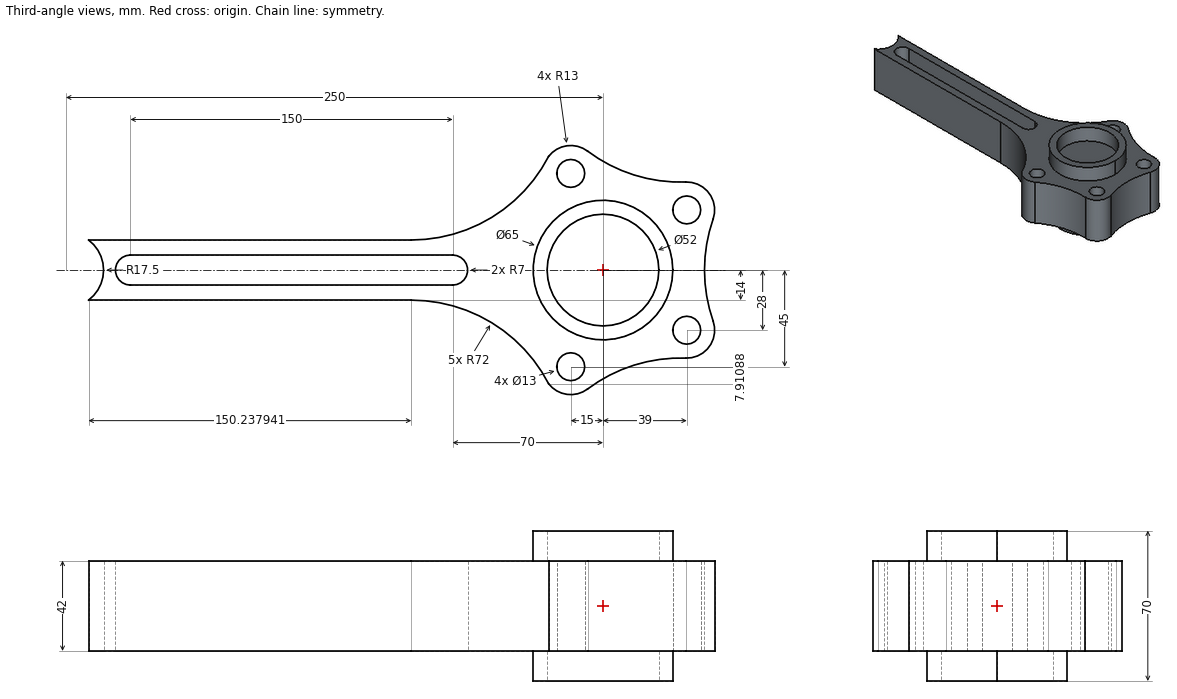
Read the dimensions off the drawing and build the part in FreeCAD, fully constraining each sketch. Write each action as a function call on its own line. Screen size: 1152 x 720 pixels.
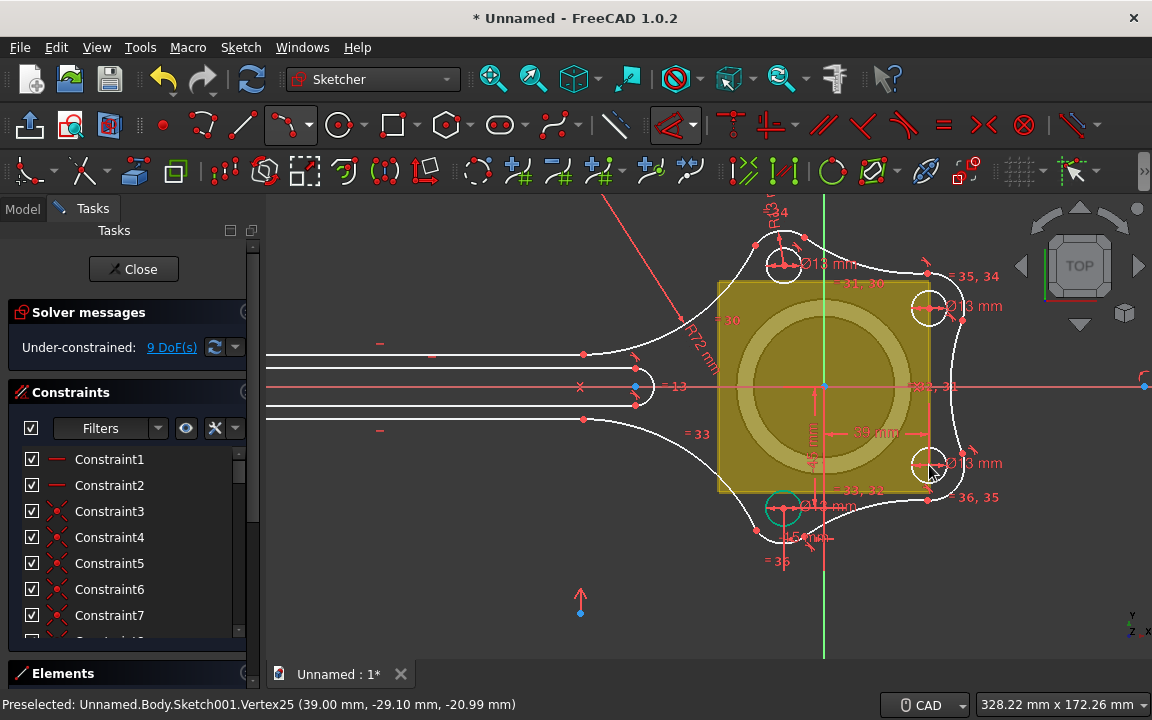
click(696, 126)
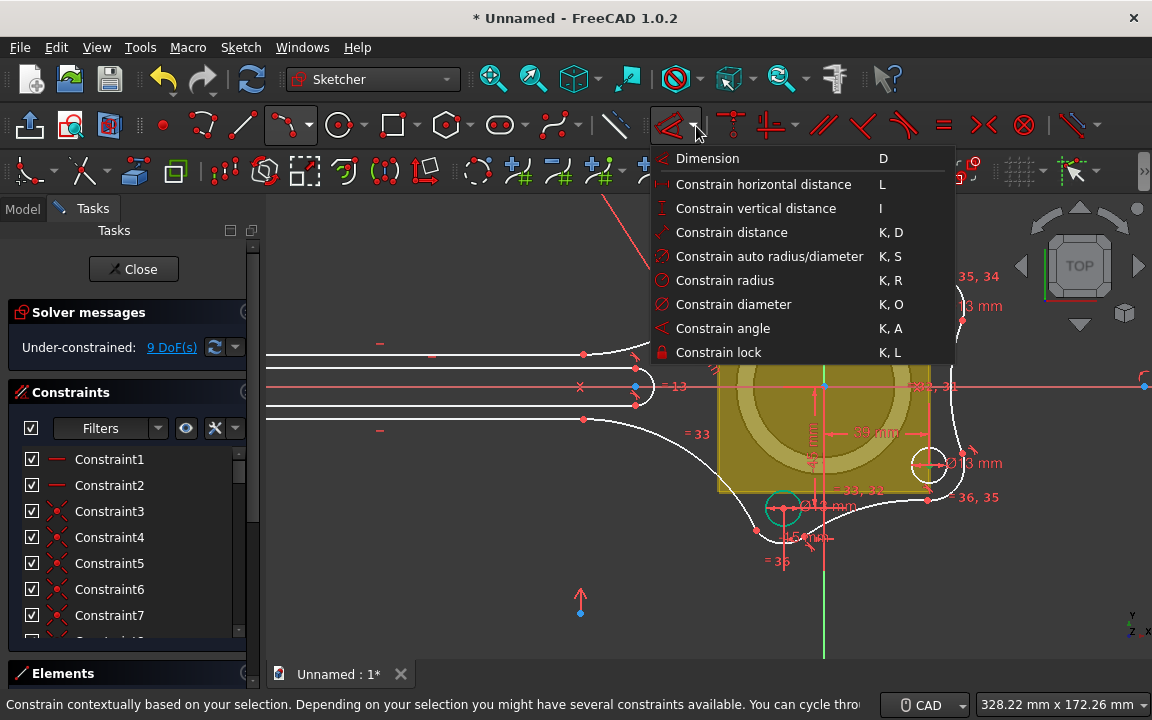
click(803, 208)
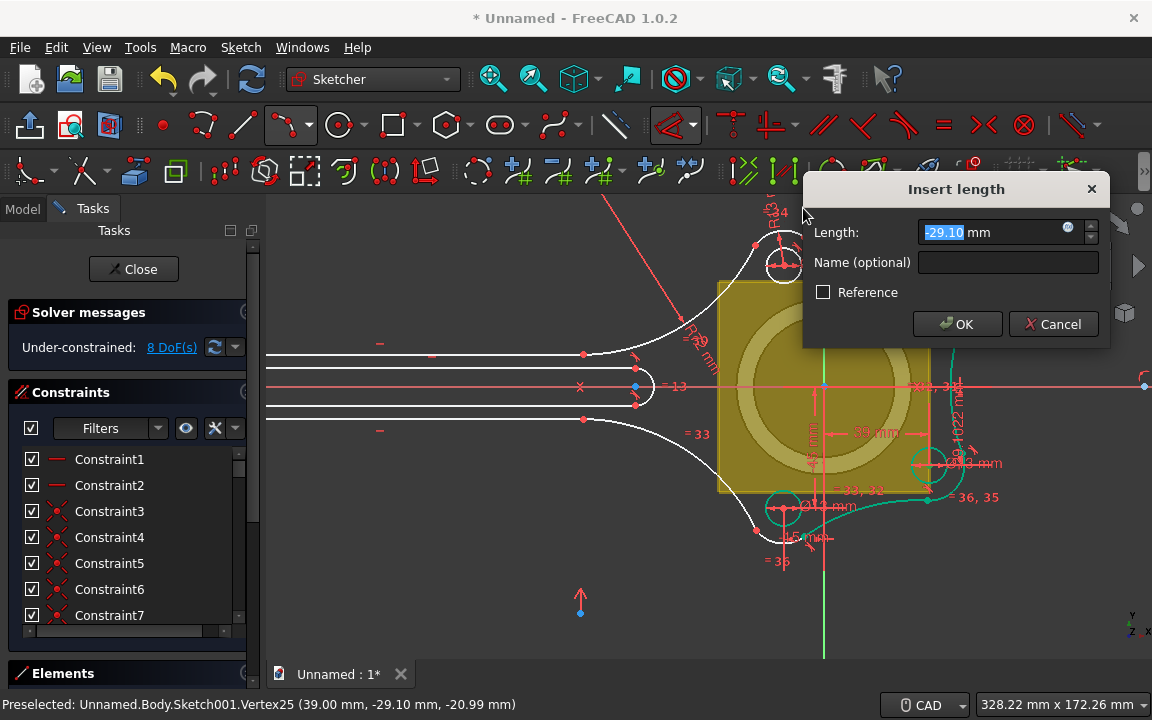
text(-28)
key(Return)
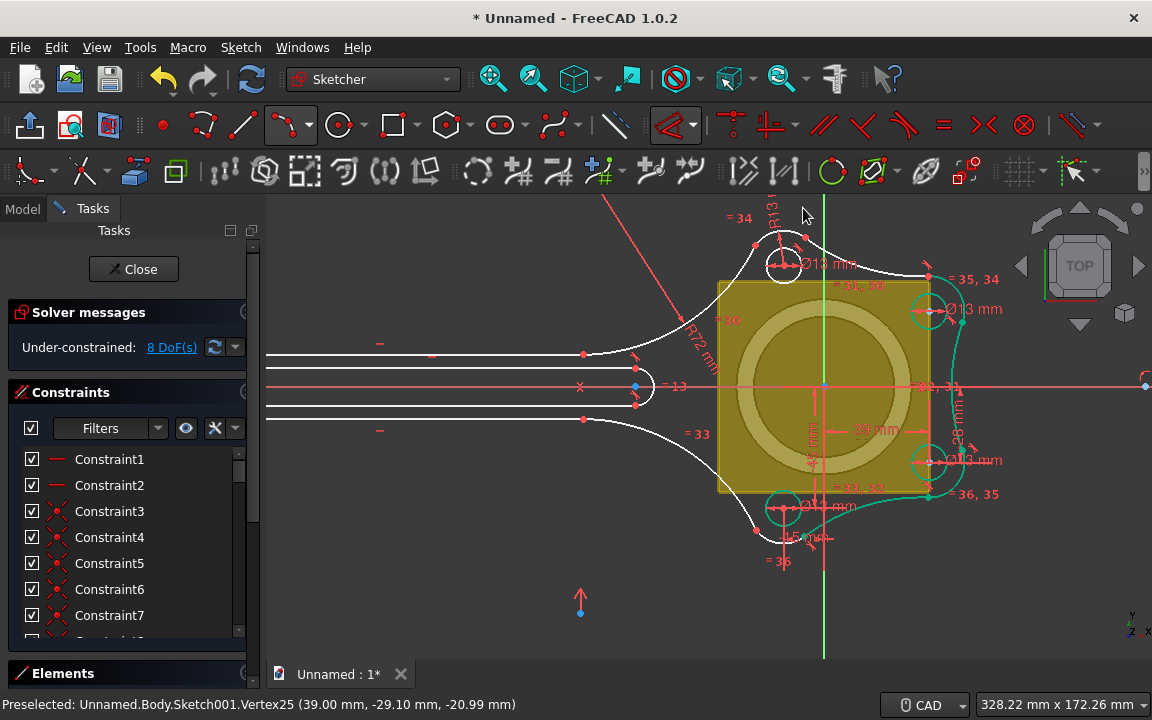
click(784, 266)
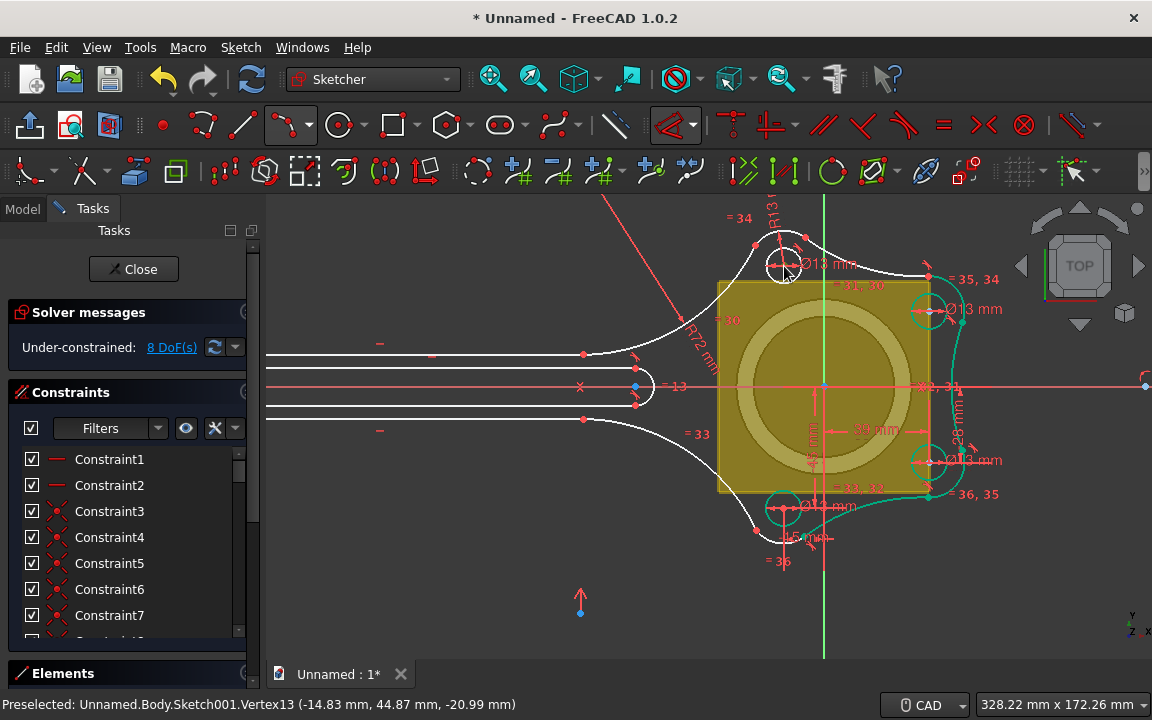
key(l)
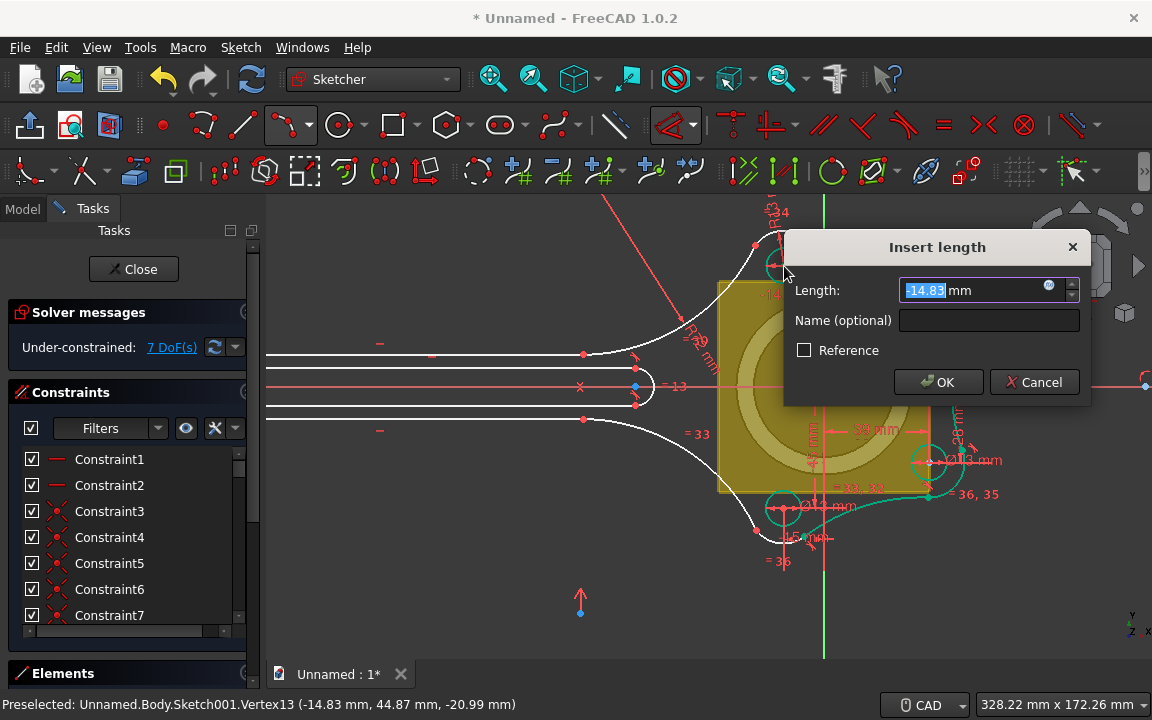
text(-15)
key(Return)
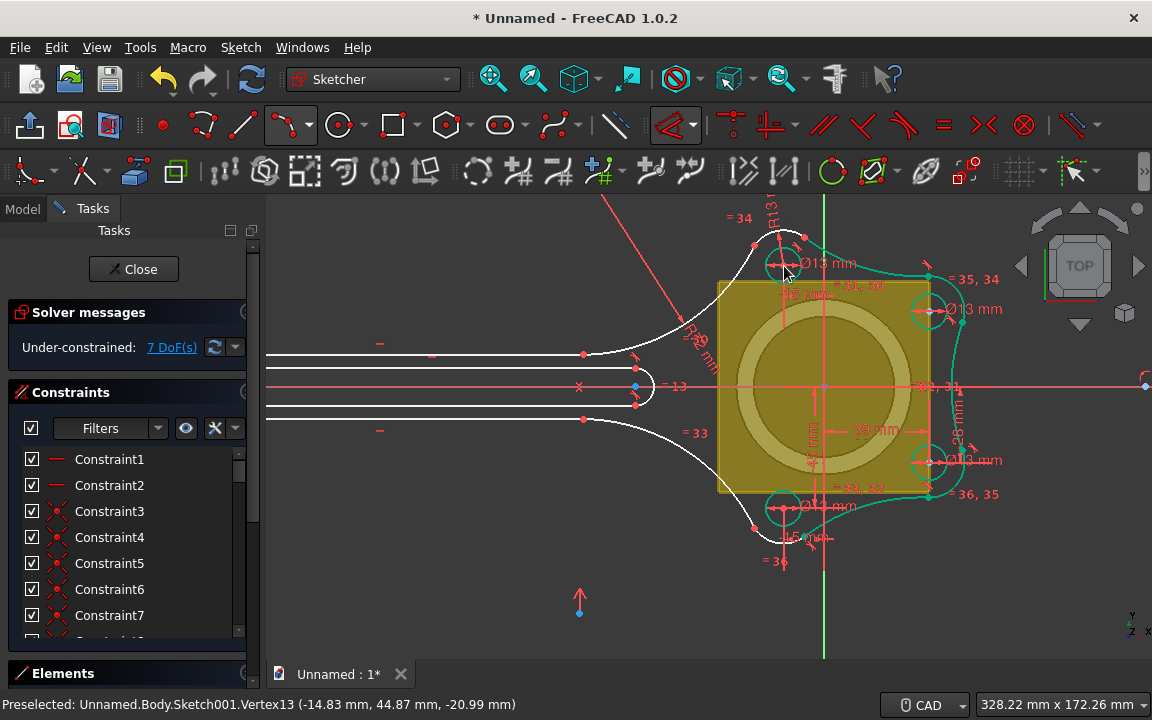
click(352, 368)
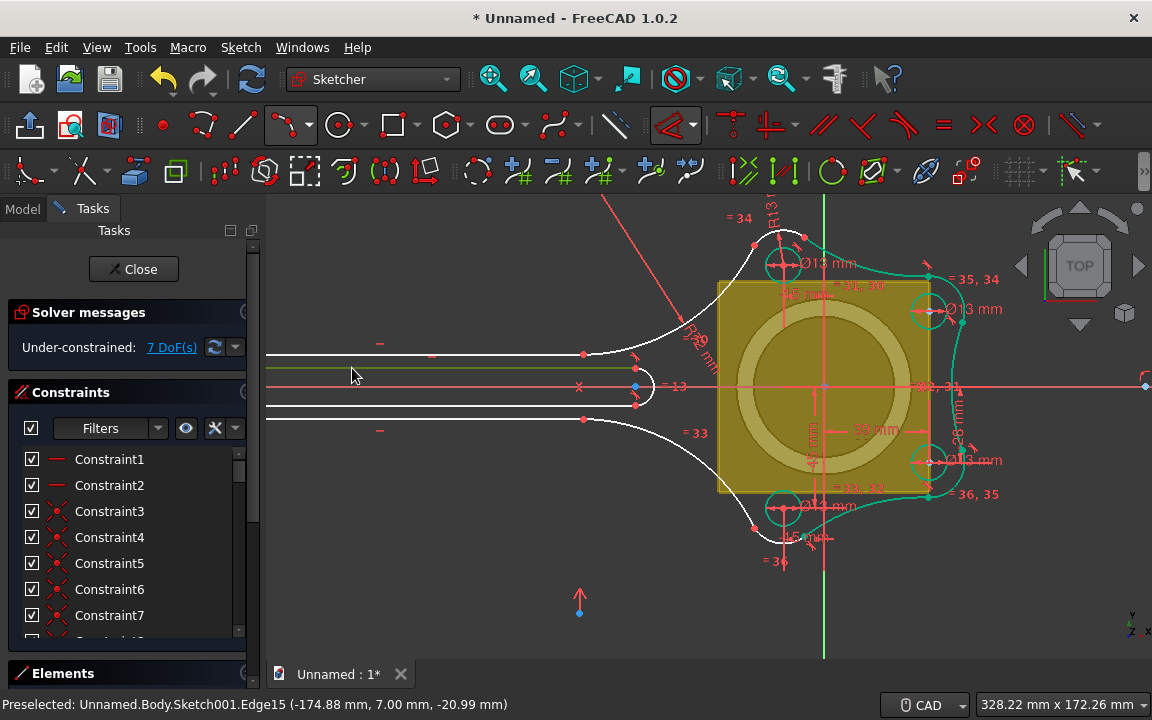
key(l)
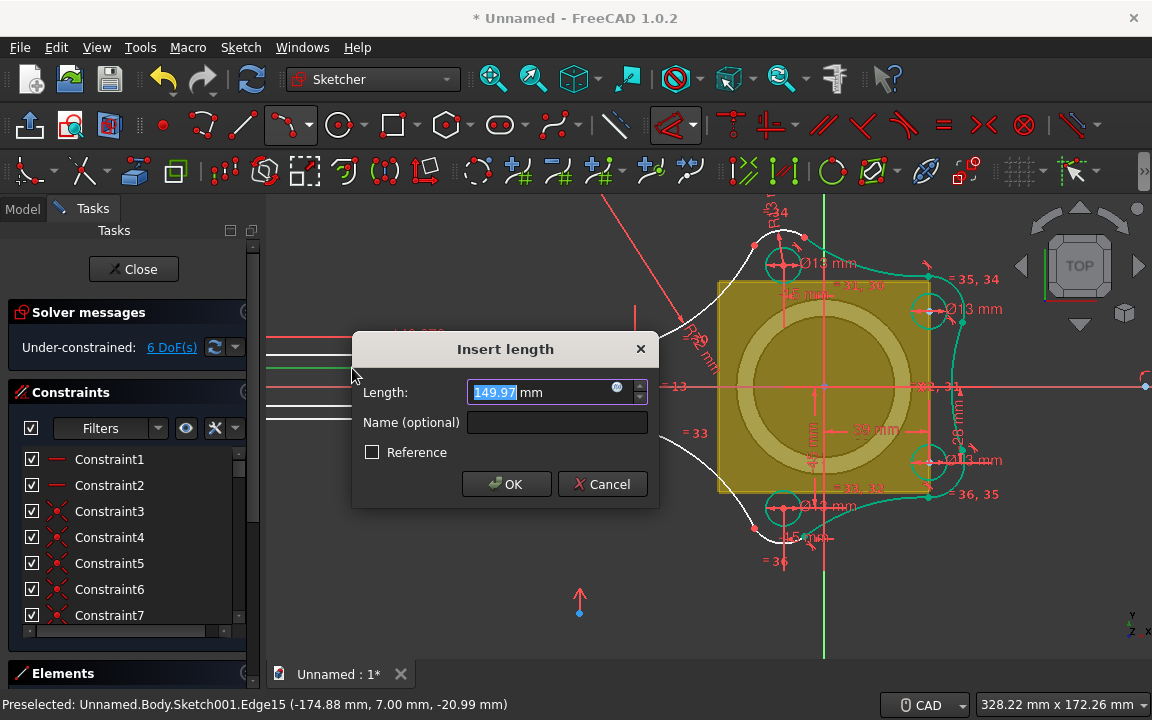
text(150)
key(Return)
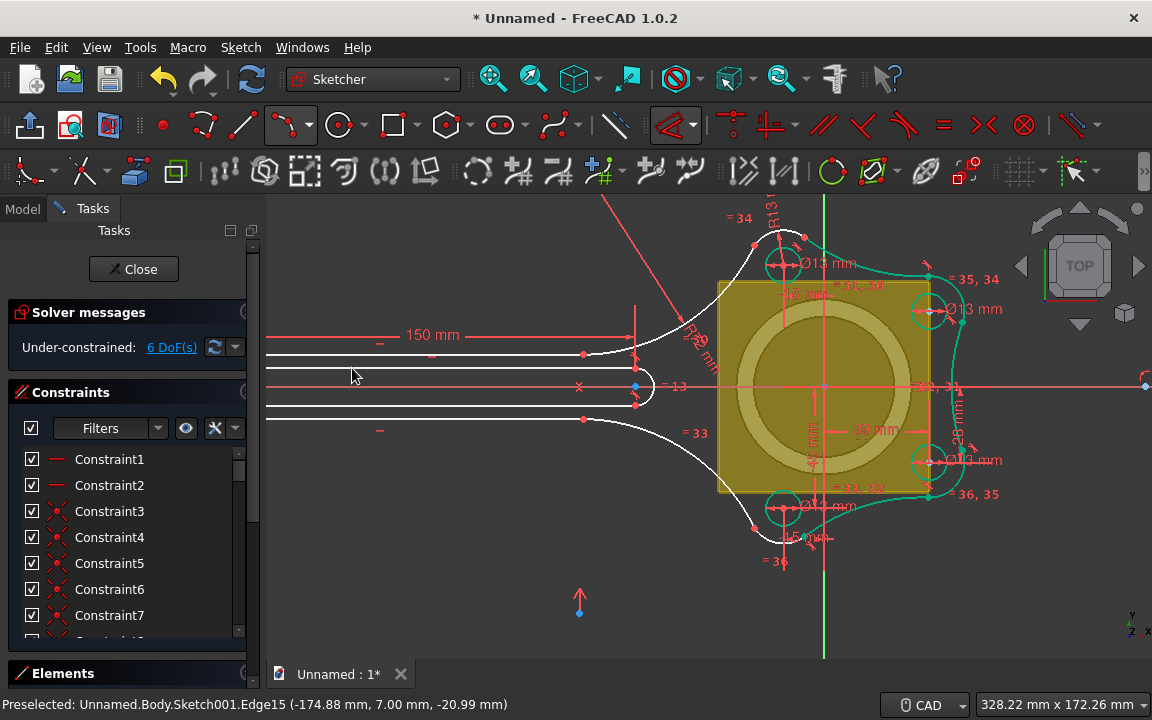
click(584, 419)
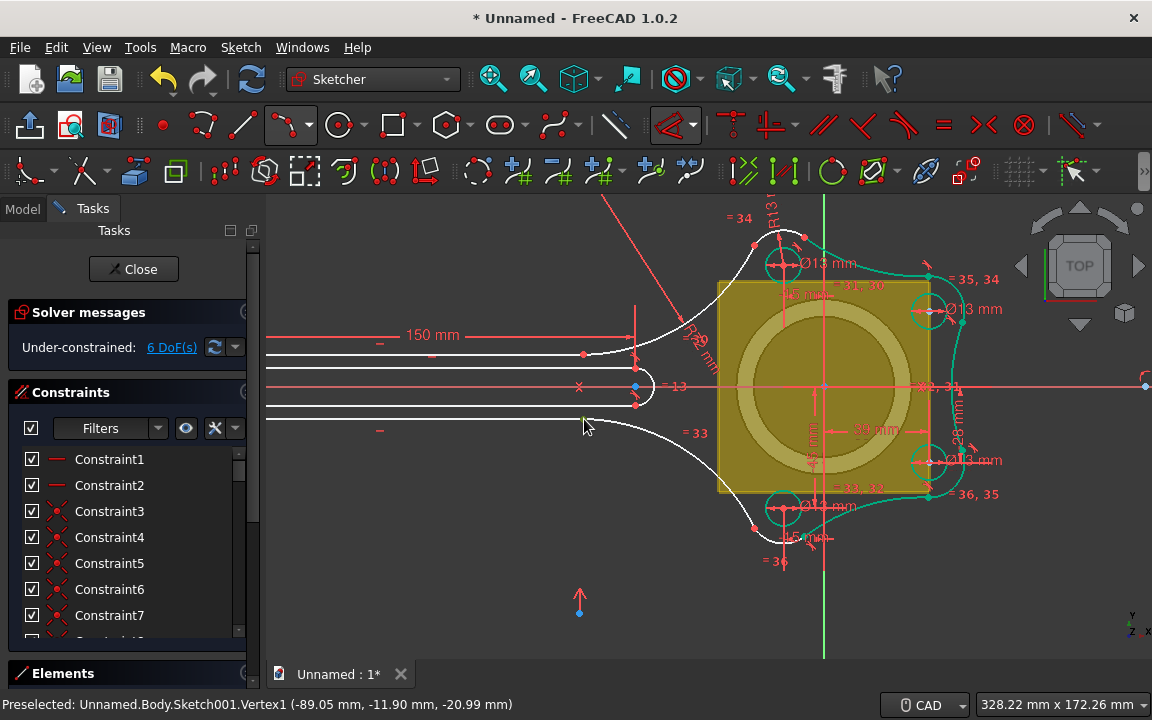
click(696, 126)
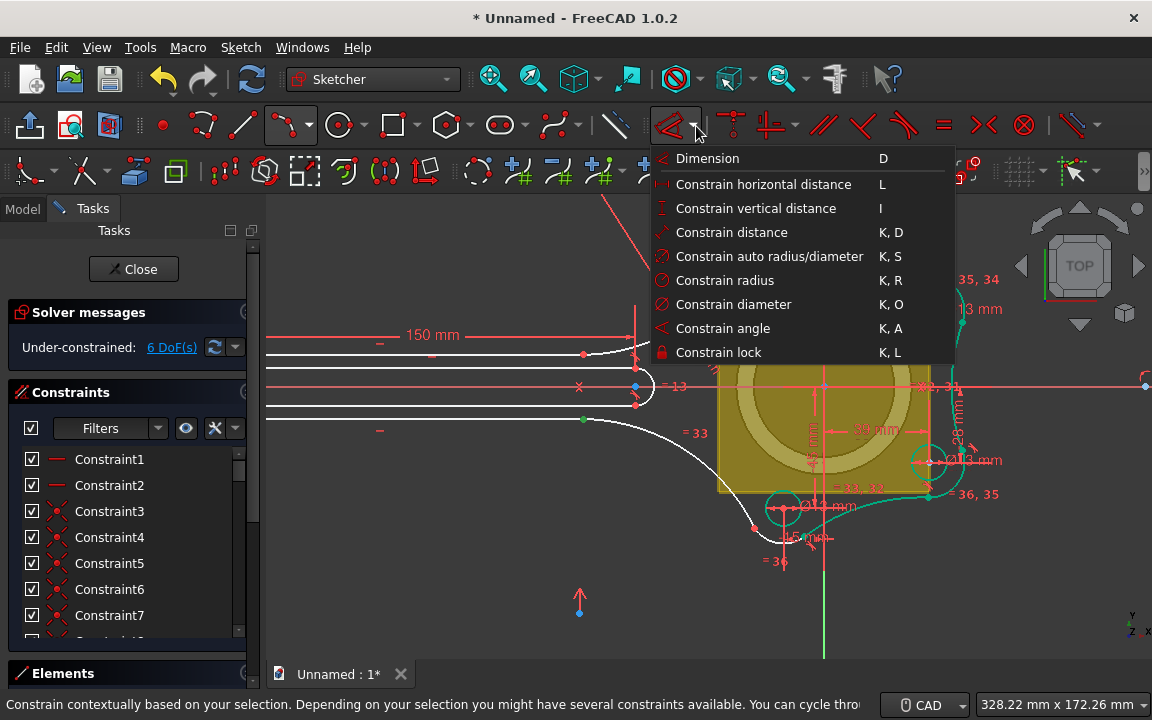
click(803, 208)